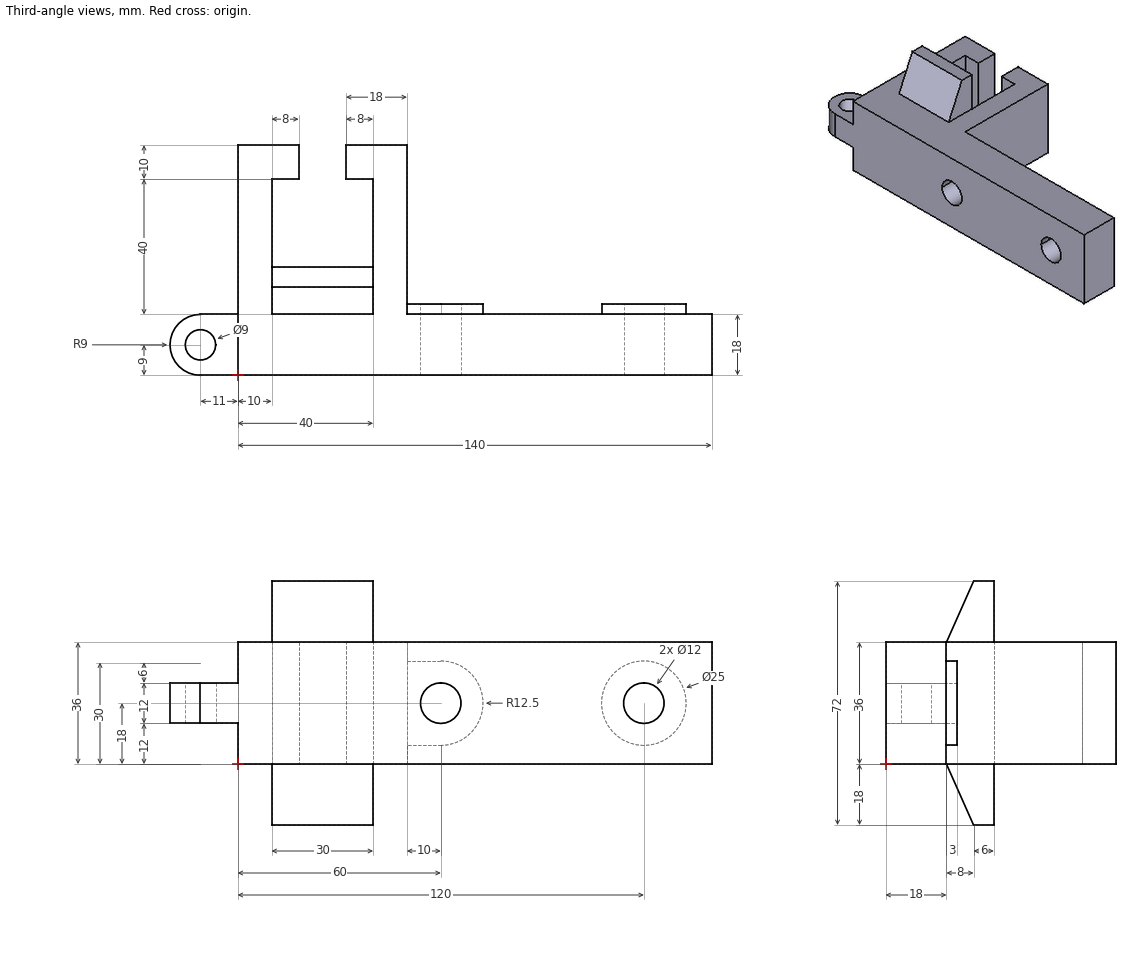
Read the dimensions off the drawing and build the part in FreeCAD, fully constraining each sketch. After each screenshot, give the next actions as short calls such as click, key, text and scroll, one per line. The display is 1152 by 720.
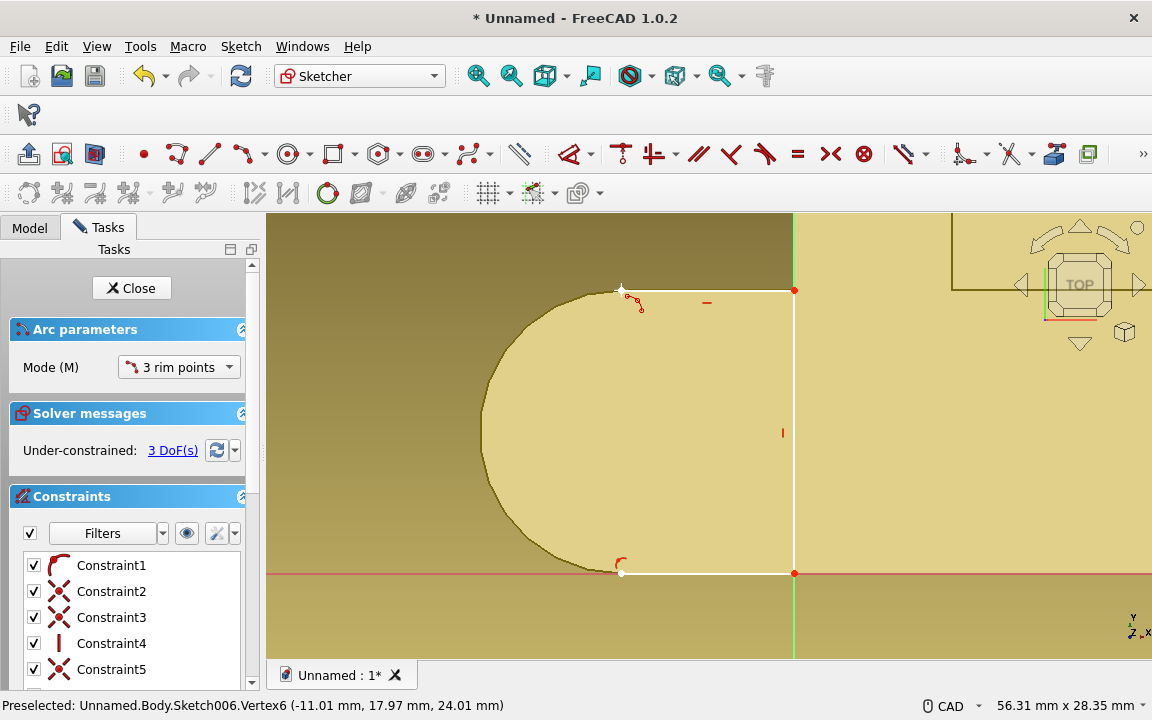
click(621, 291)
click(621, 574)
click(480, 432)
key(Escape)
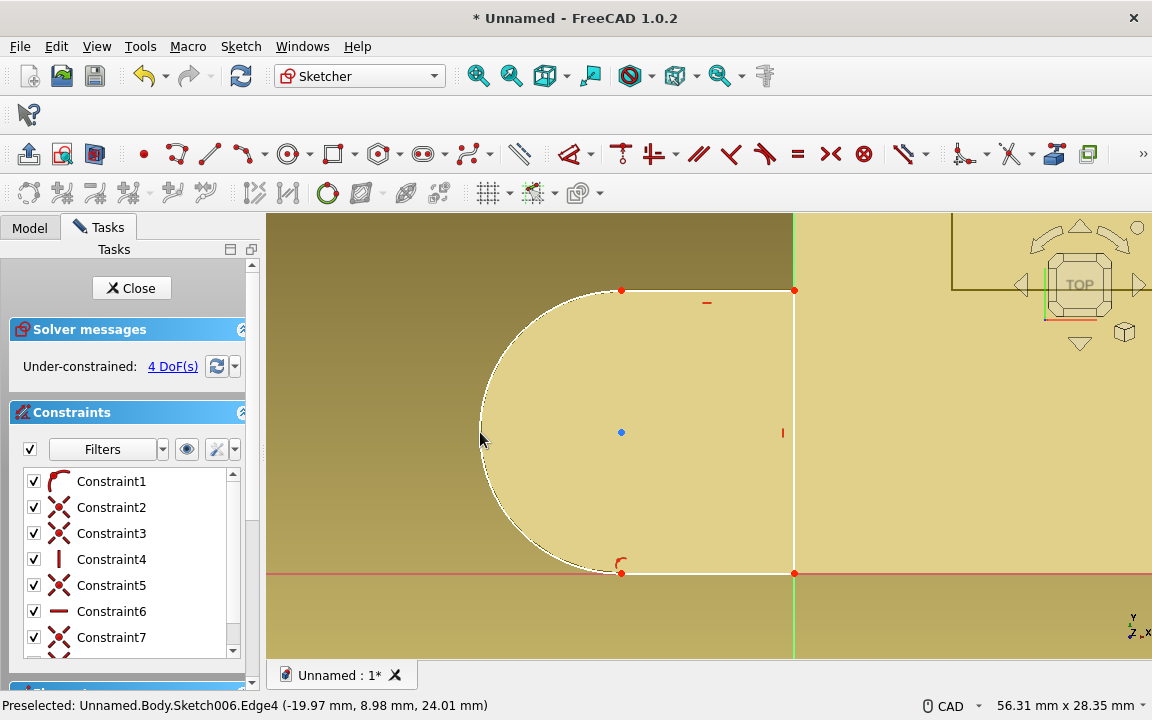
click(673, 574)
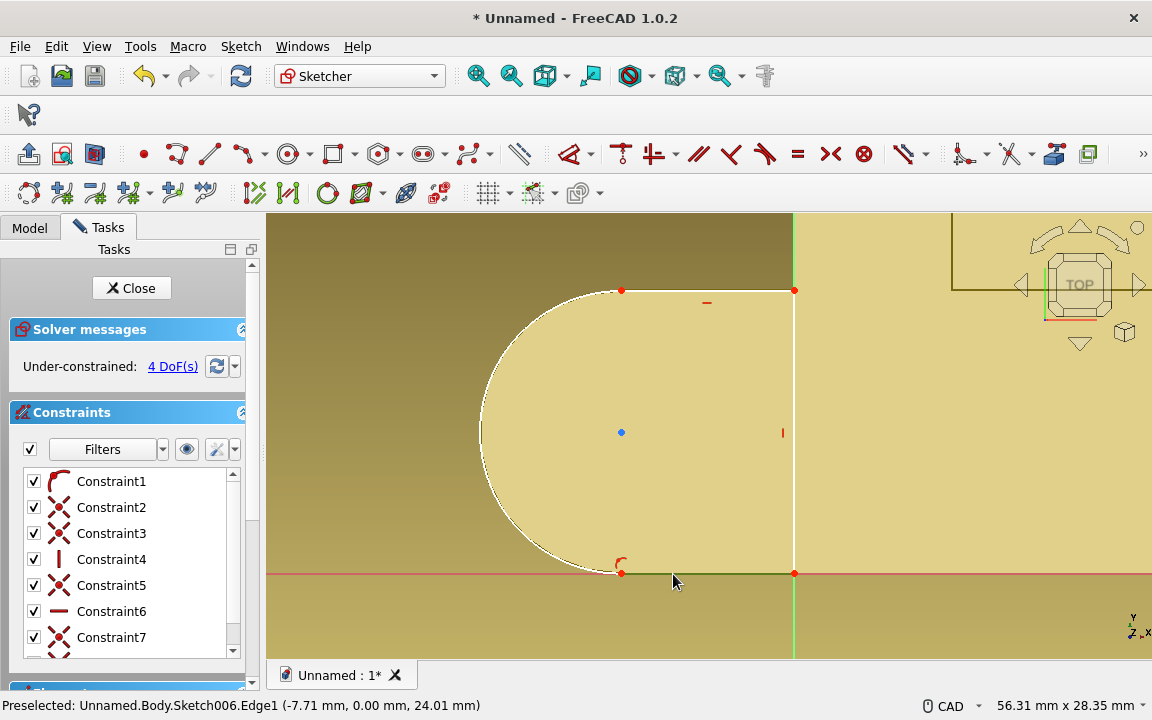
click(507, 349)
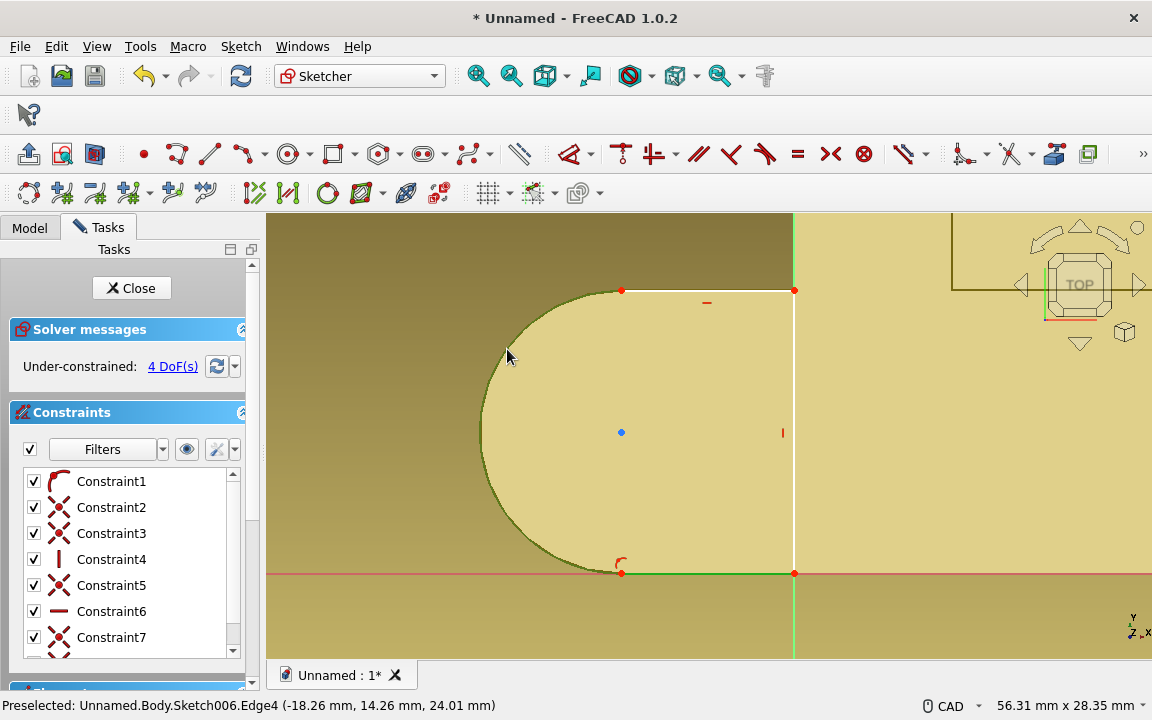
click(765, 154)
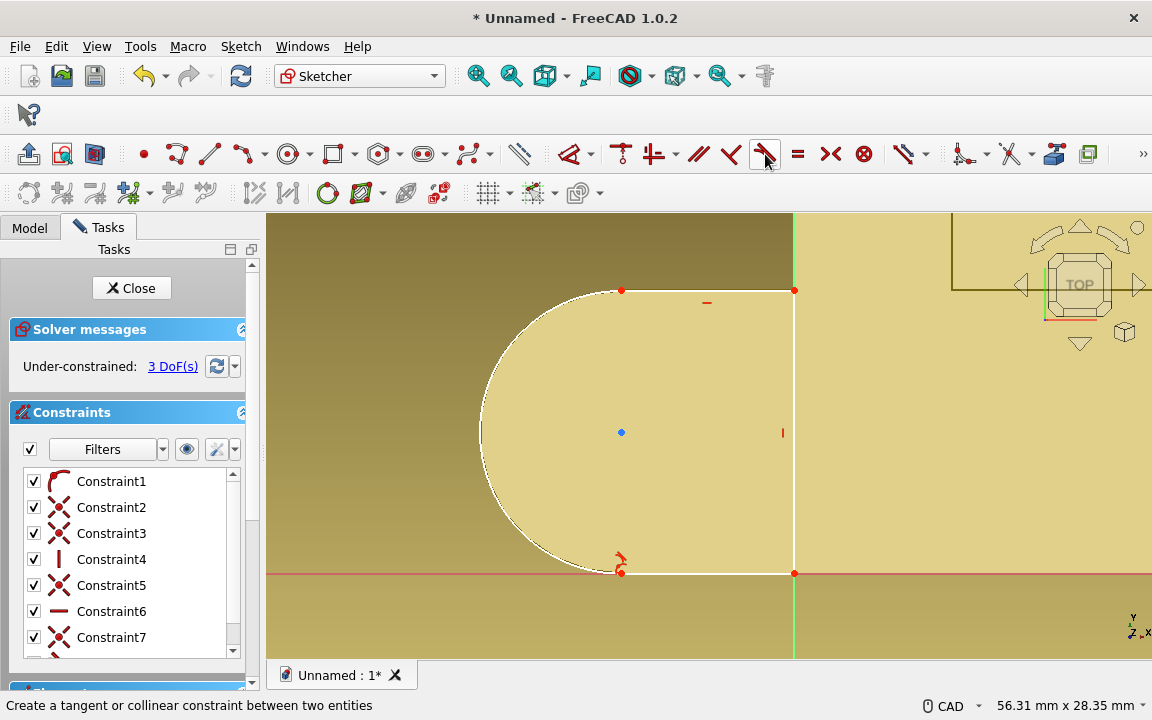
click(742, 291)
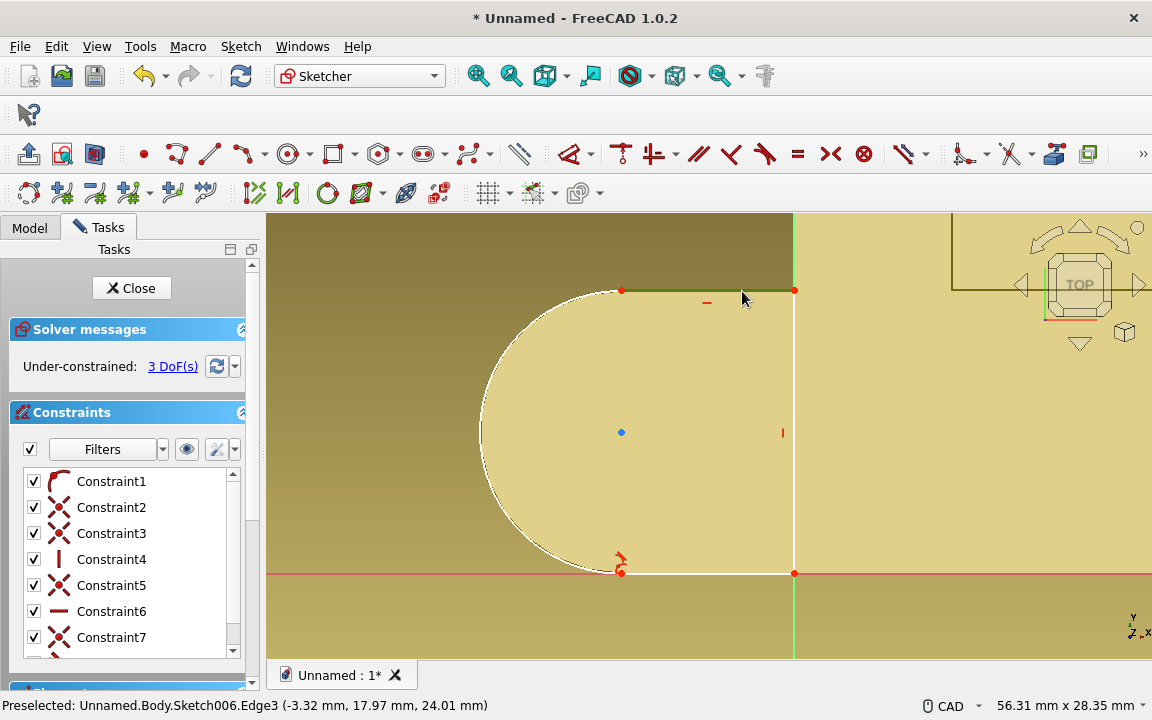
click(507, 349)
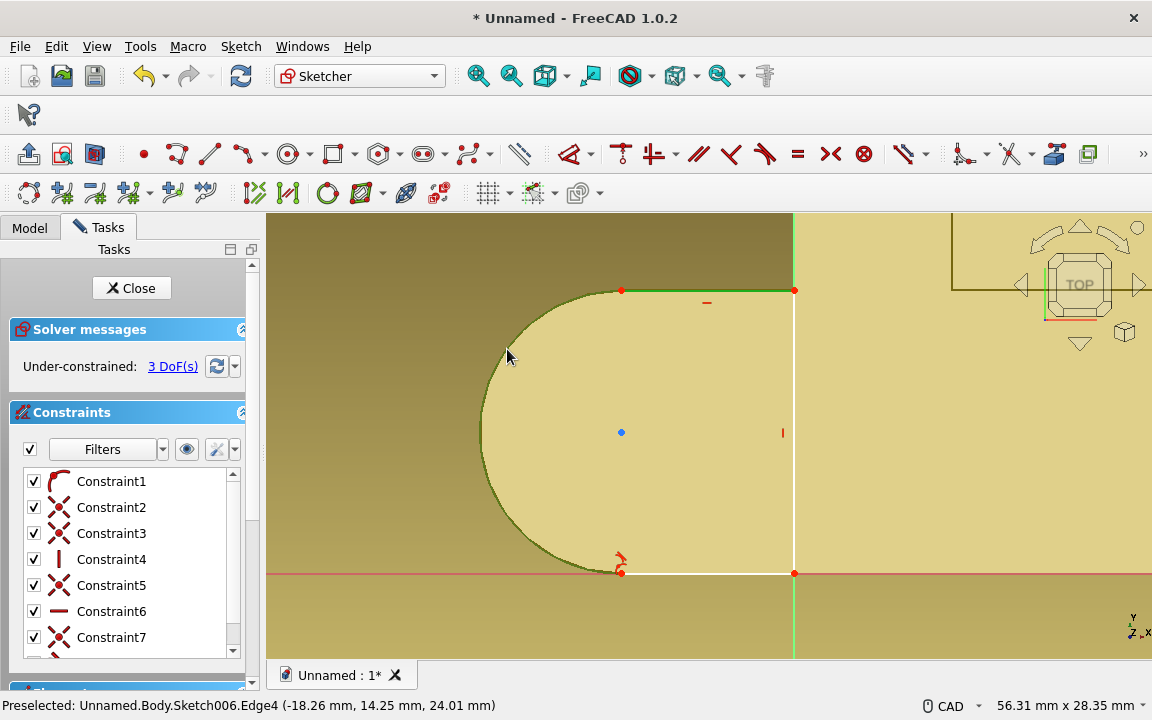
click(765, 154)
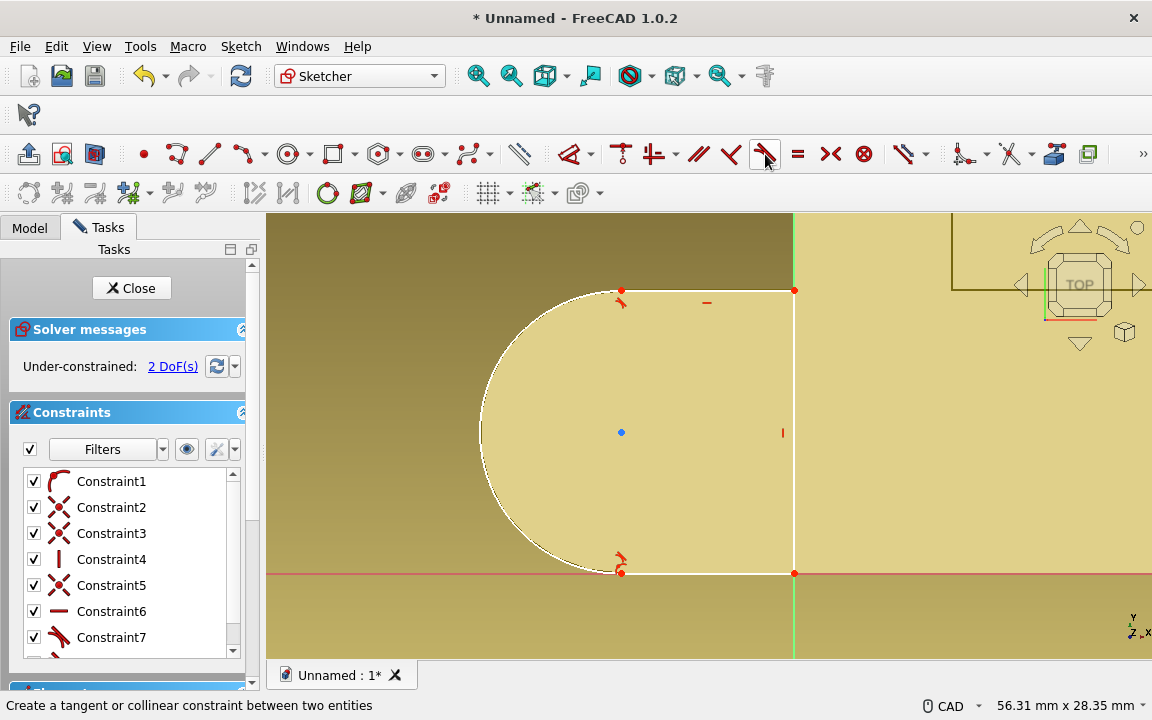
click(568, 154)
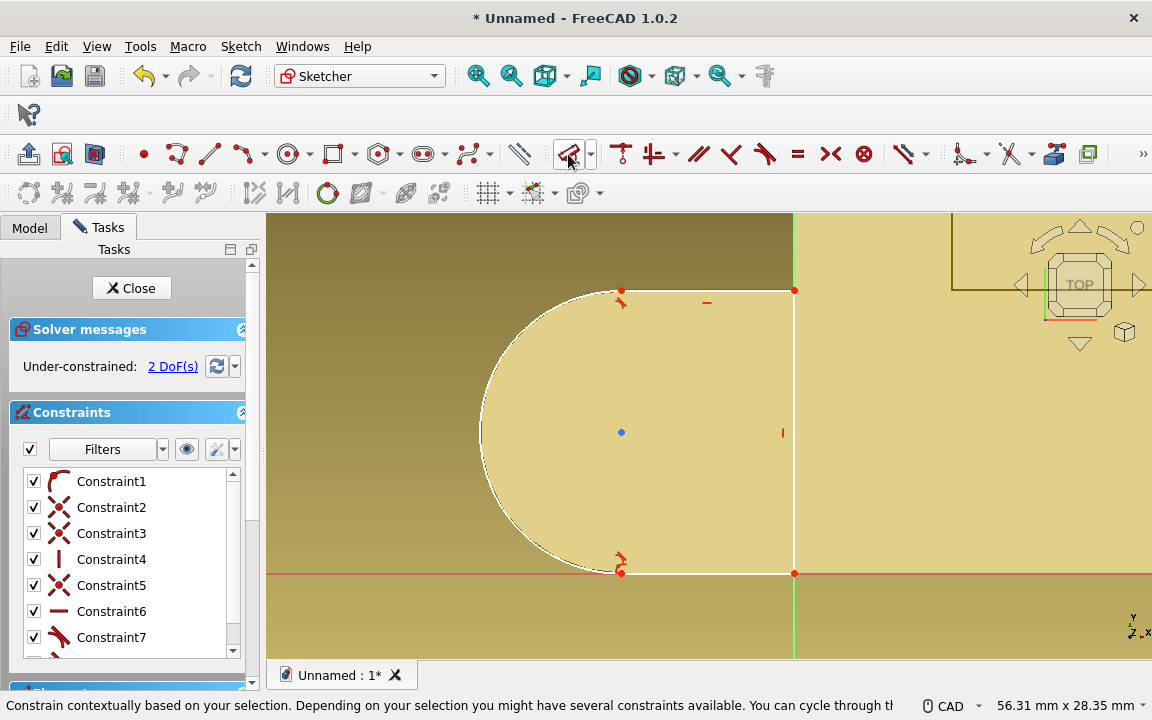
click(507, 349)
click(481, 330)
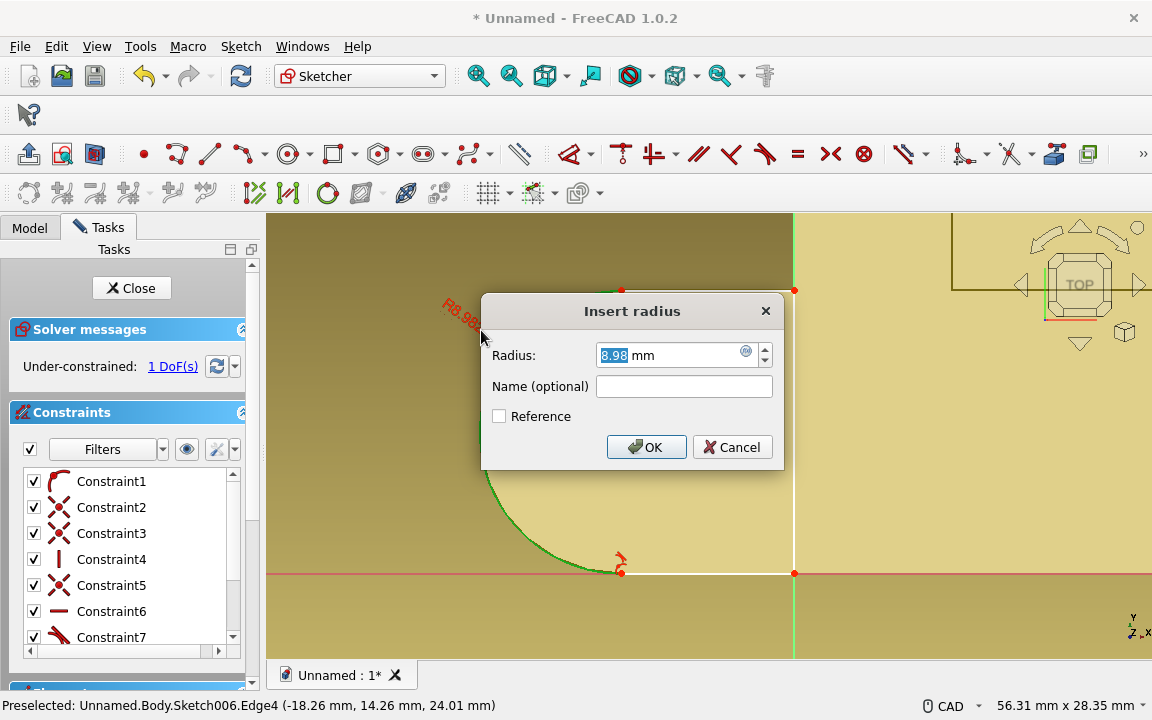
text(9)
key(Return)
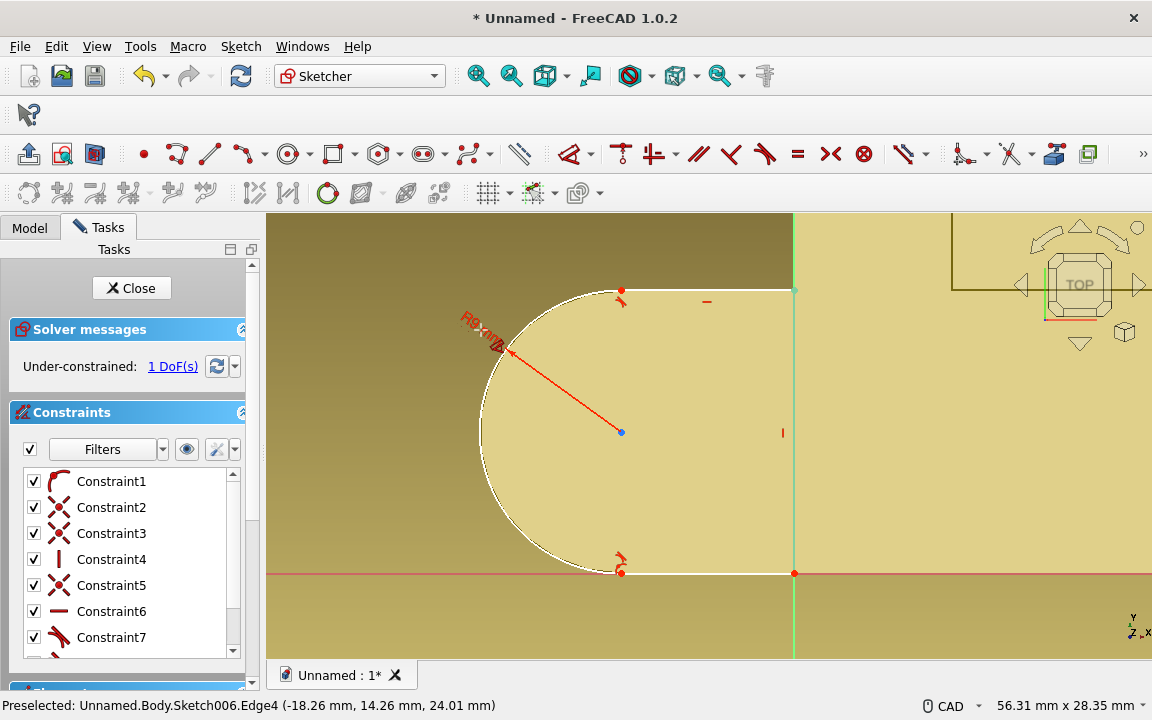
click(673, 574)
click(708, 608)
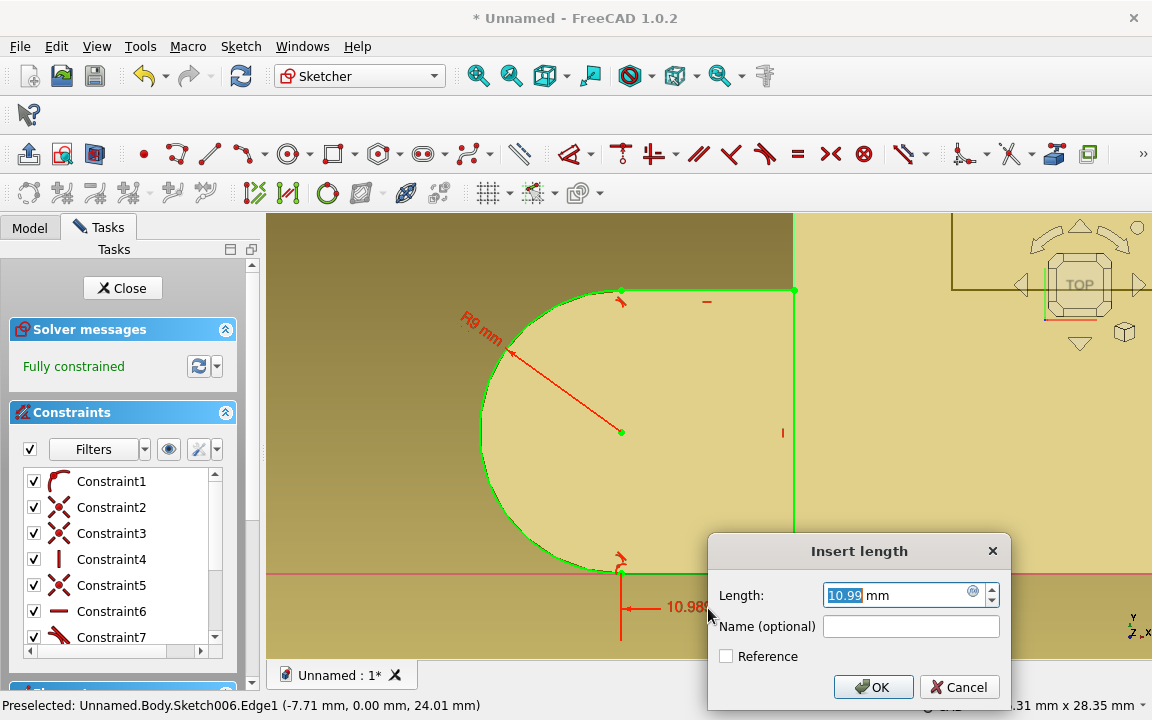
text(11)
key(Return)
key(Escape)